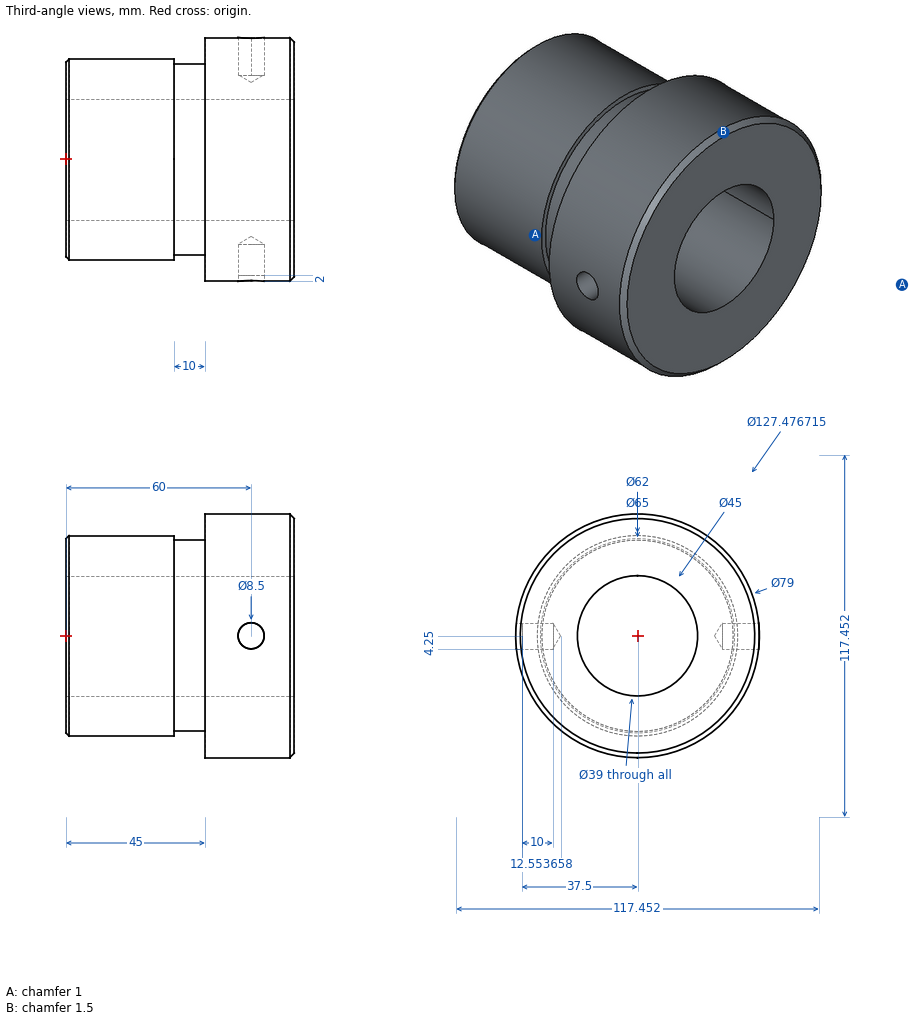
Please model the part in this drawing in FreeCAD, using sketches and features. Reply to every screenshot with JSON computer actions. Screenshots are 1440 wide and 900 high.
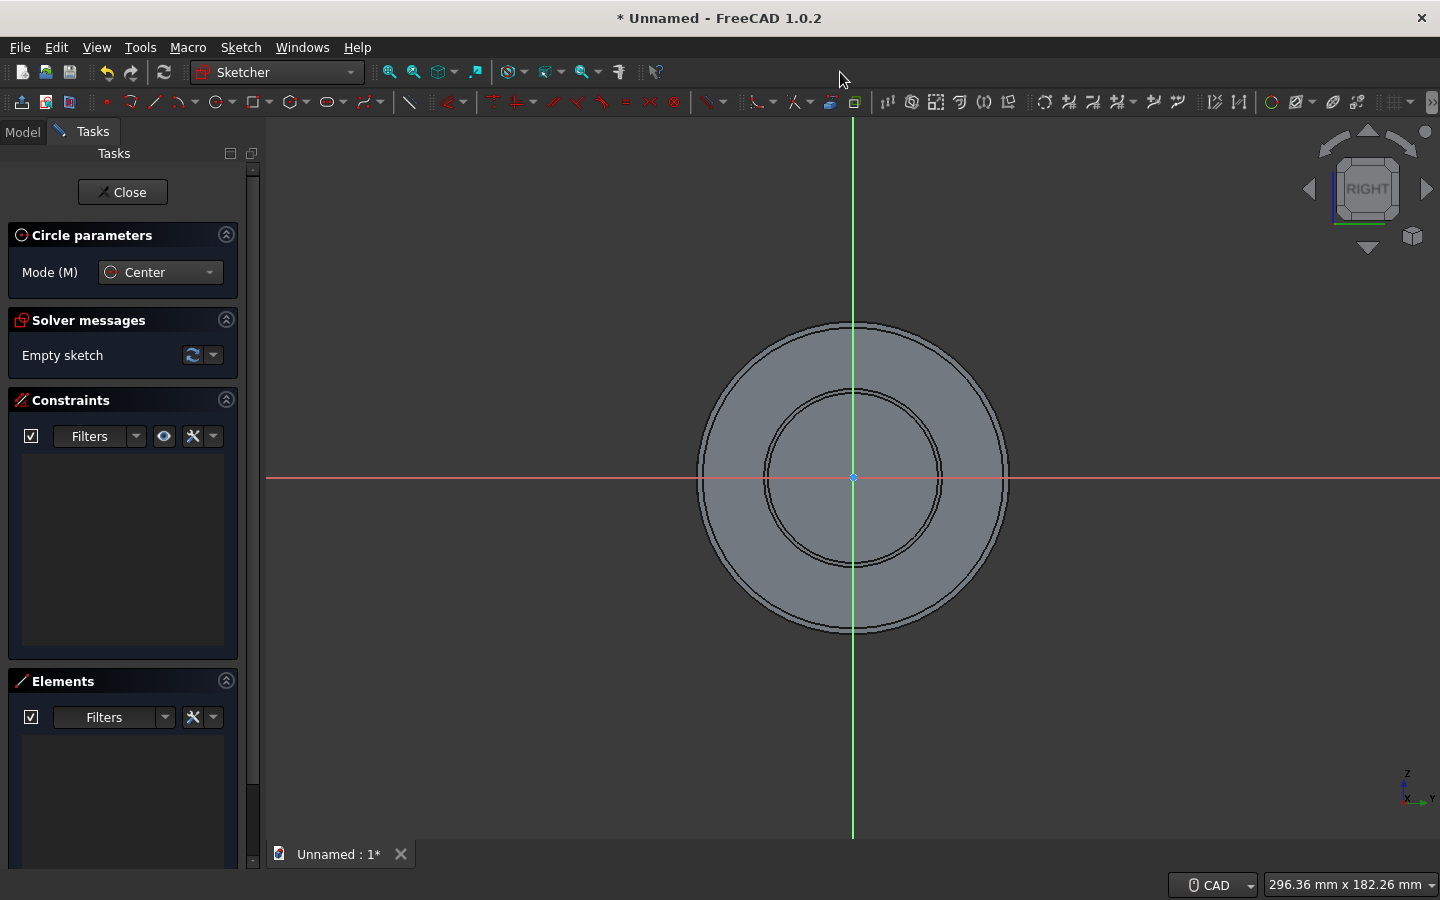
{"action": "left_click", "coordinate": [853, 478]}
{"action": "mouse_move", "coordinate": [1032, 299]}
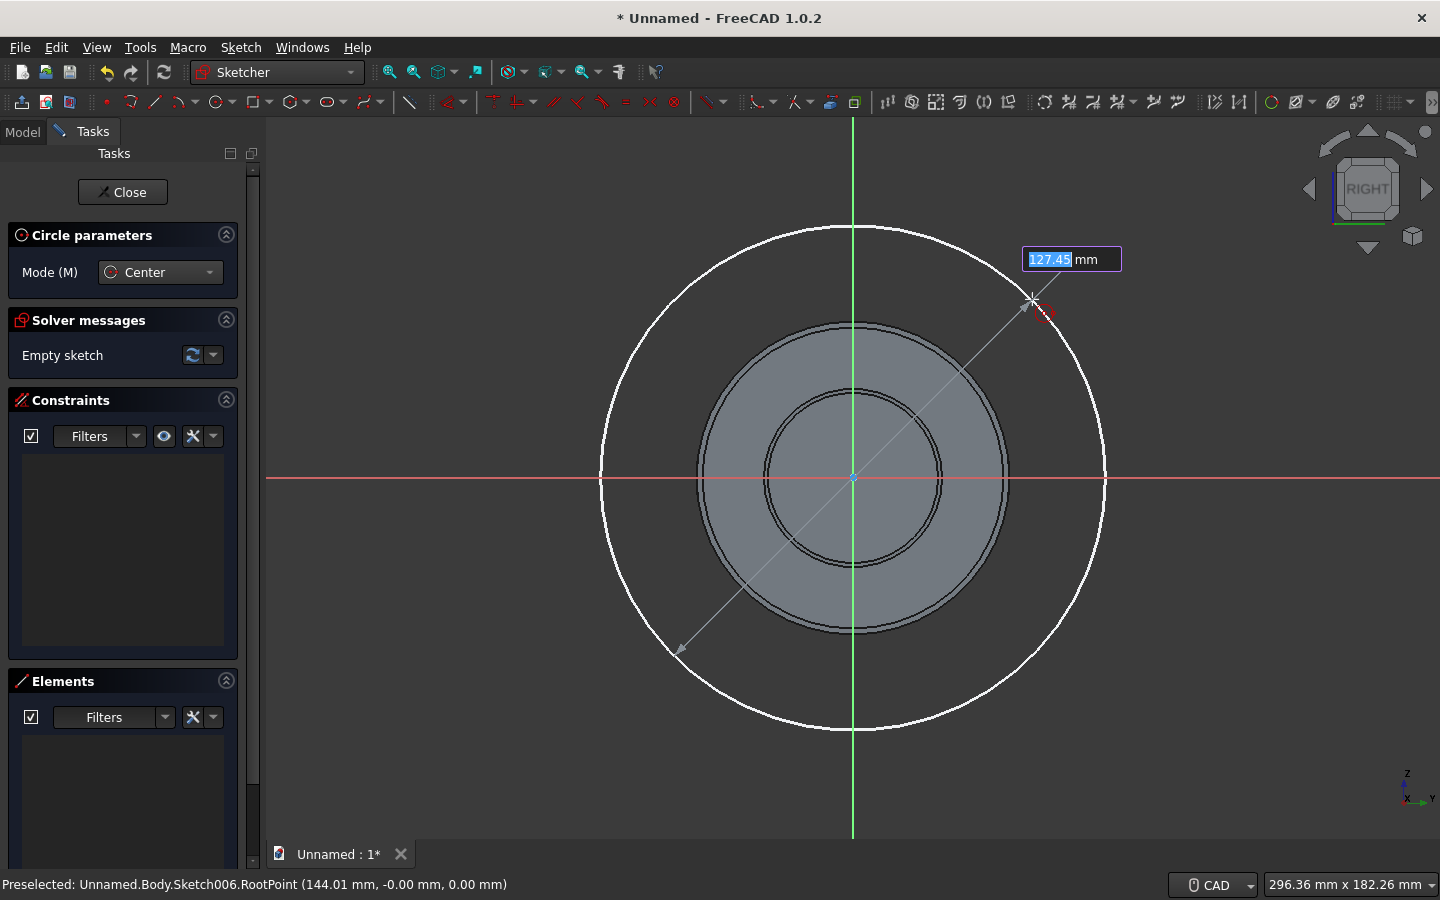
{"action": "type", "text": "127.476715"}
{"action": "key", "text": "Return"}
{"action": "key", "text": "Escape"}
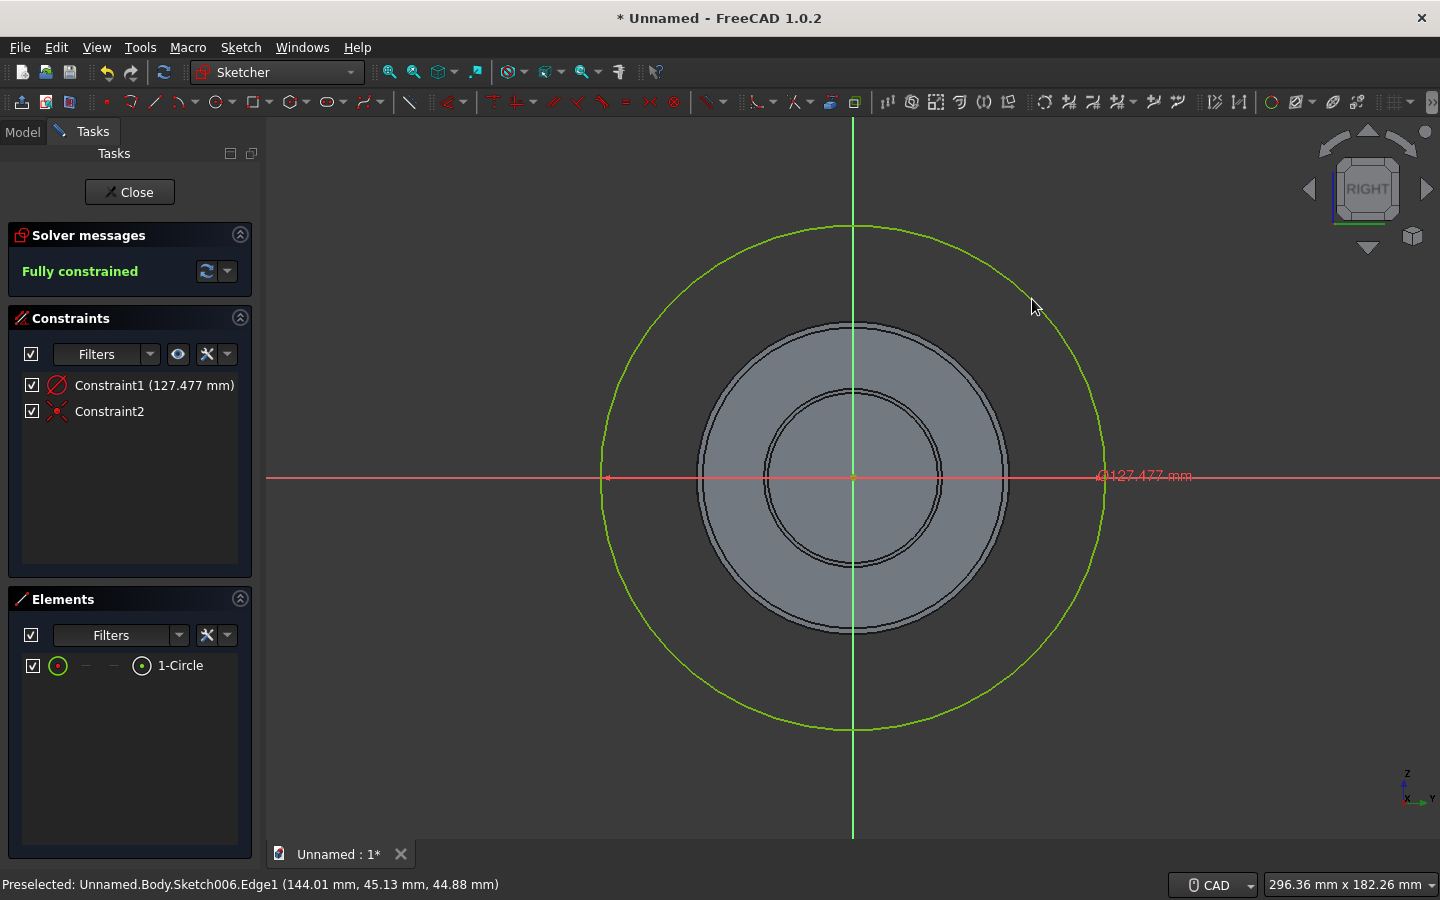
{"action": "left_click", "coordinate": [130, 192]}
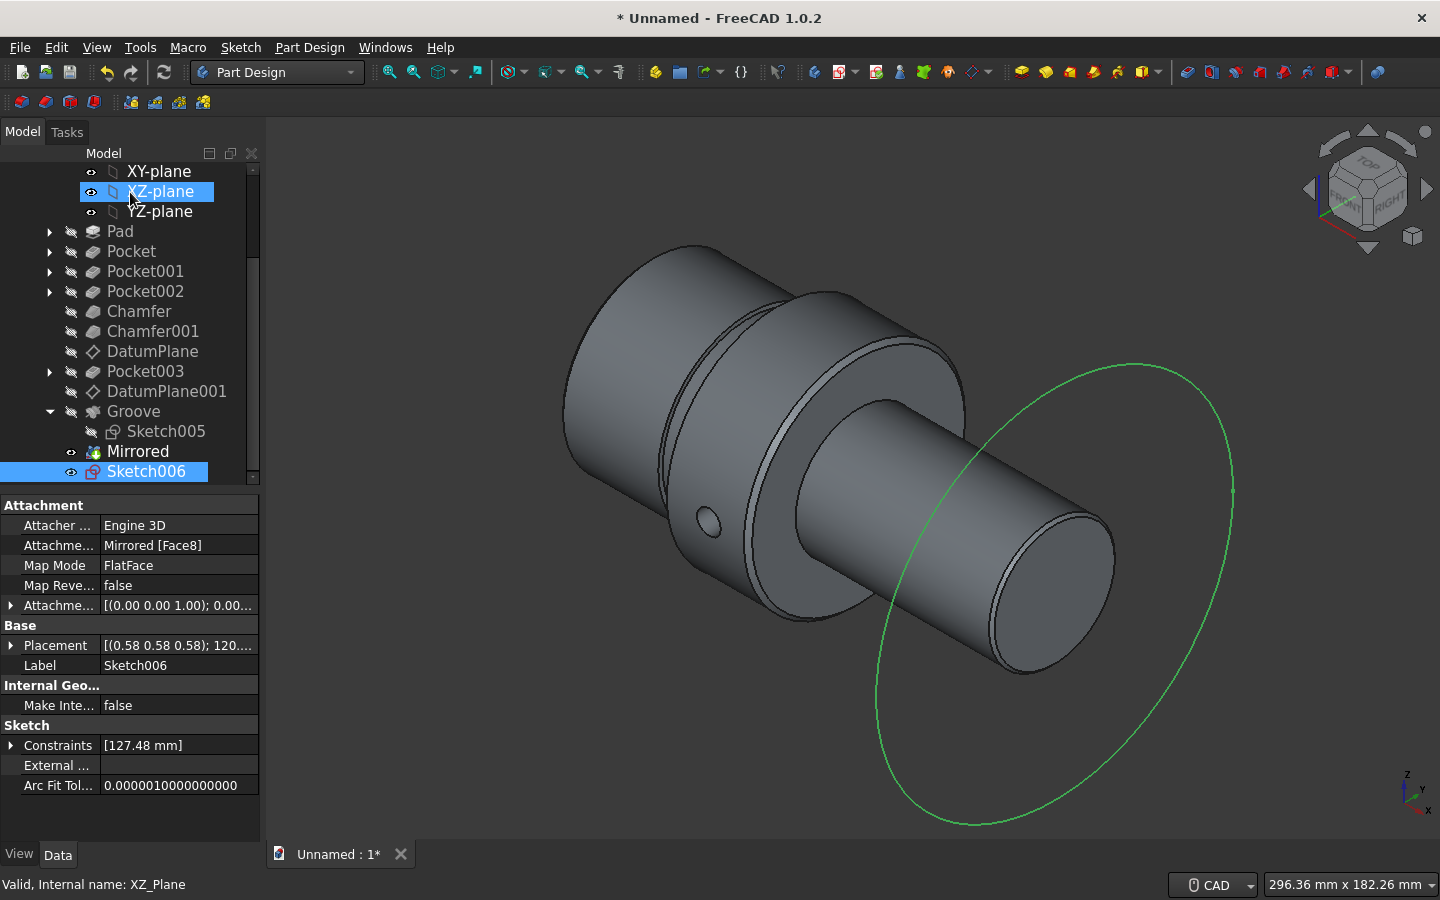
{"action": "left_click", "coordinate": [1188, 72]}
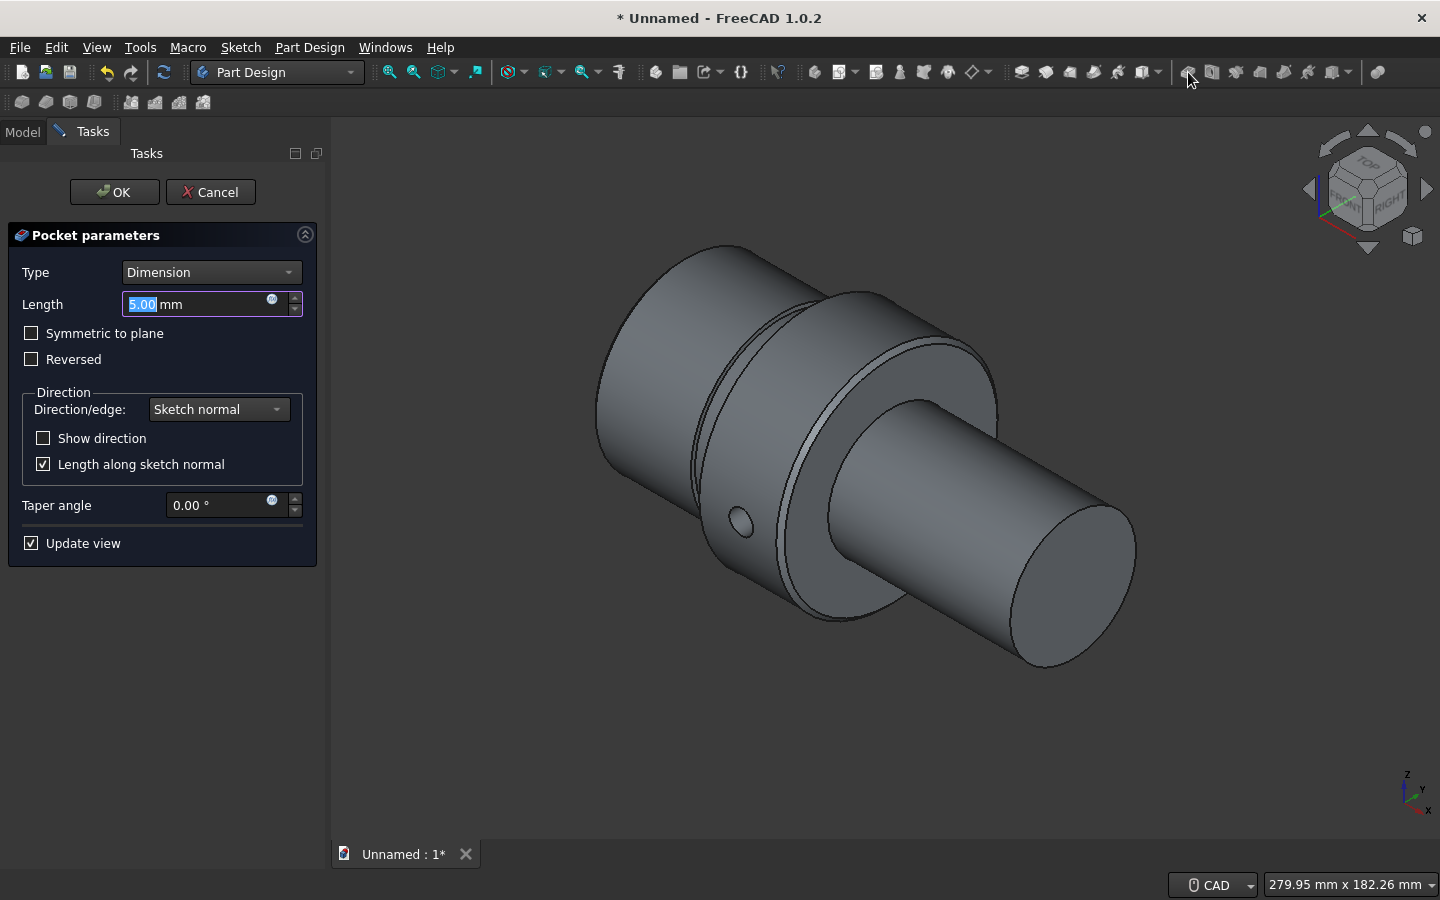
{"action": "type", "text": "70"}
{"action": "key", "text": "Tab"}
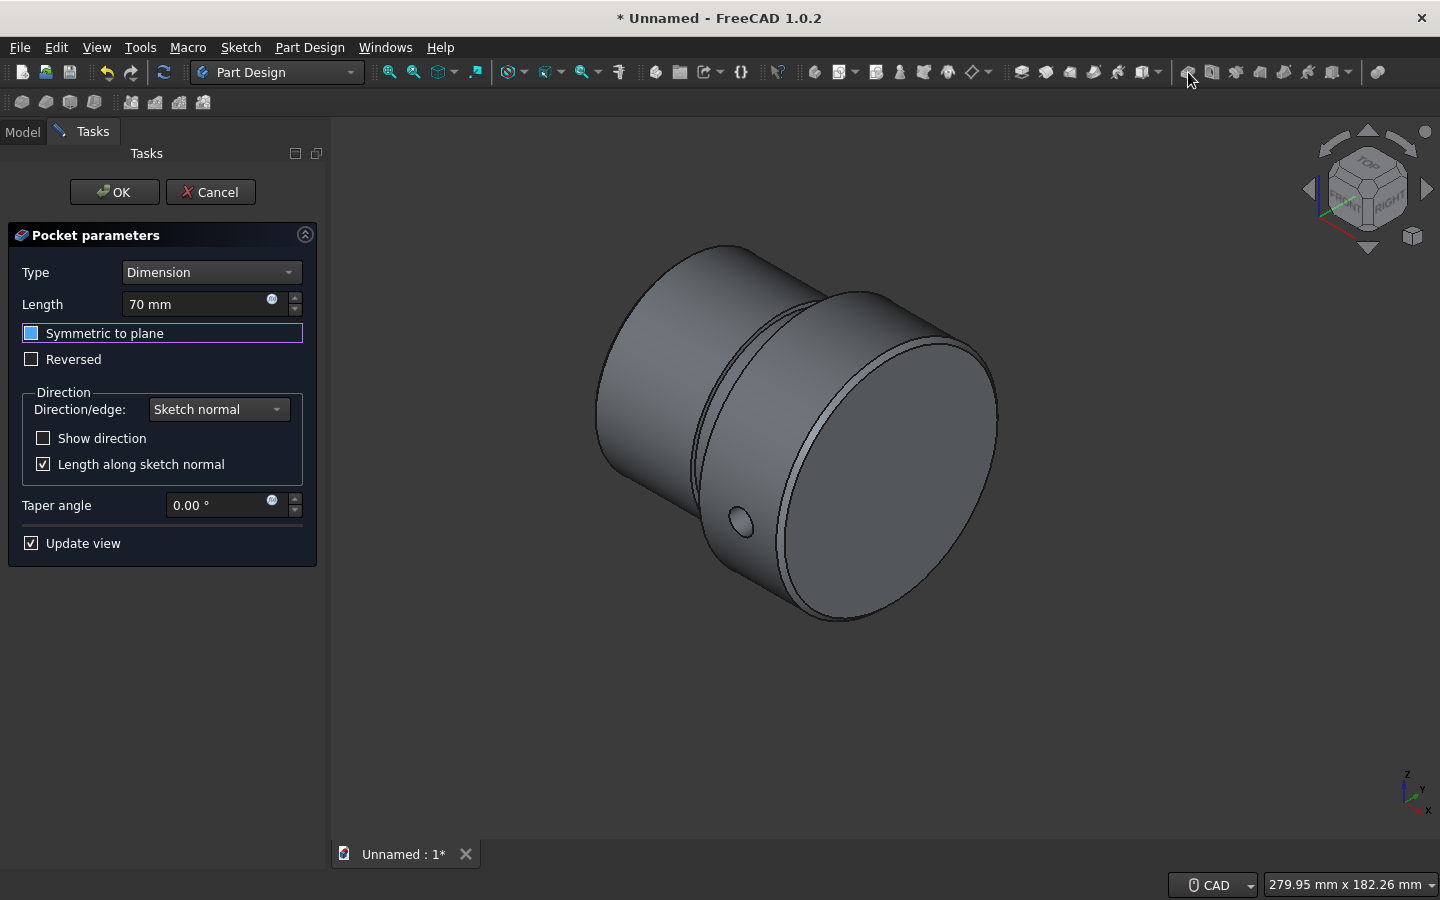
{"action": "left_click", "coordinate": [115, 192]}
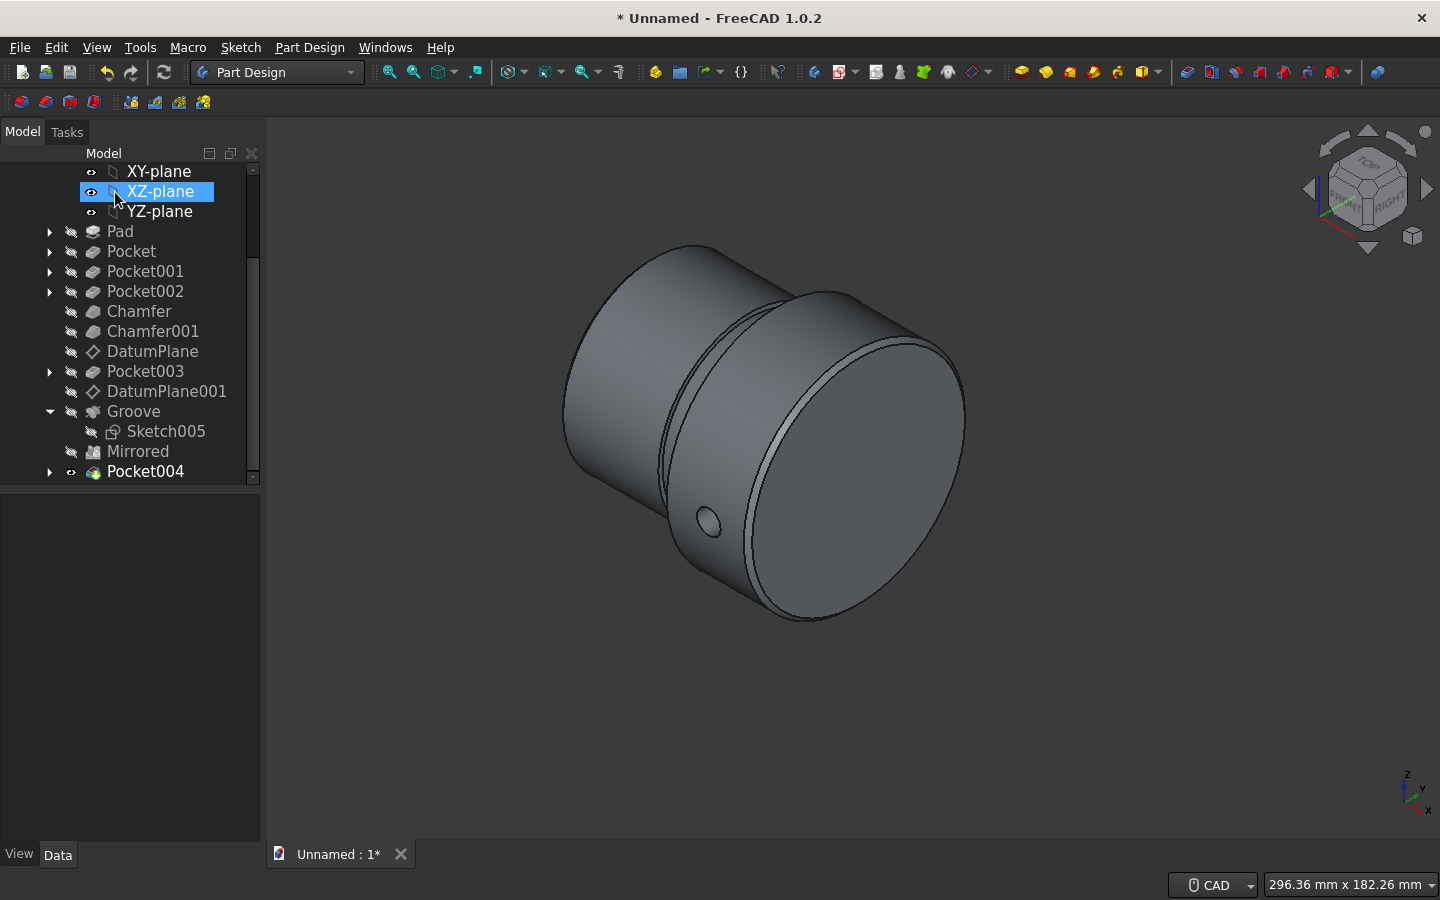
{"action": "left_click", "coordinate": [859, 480]}